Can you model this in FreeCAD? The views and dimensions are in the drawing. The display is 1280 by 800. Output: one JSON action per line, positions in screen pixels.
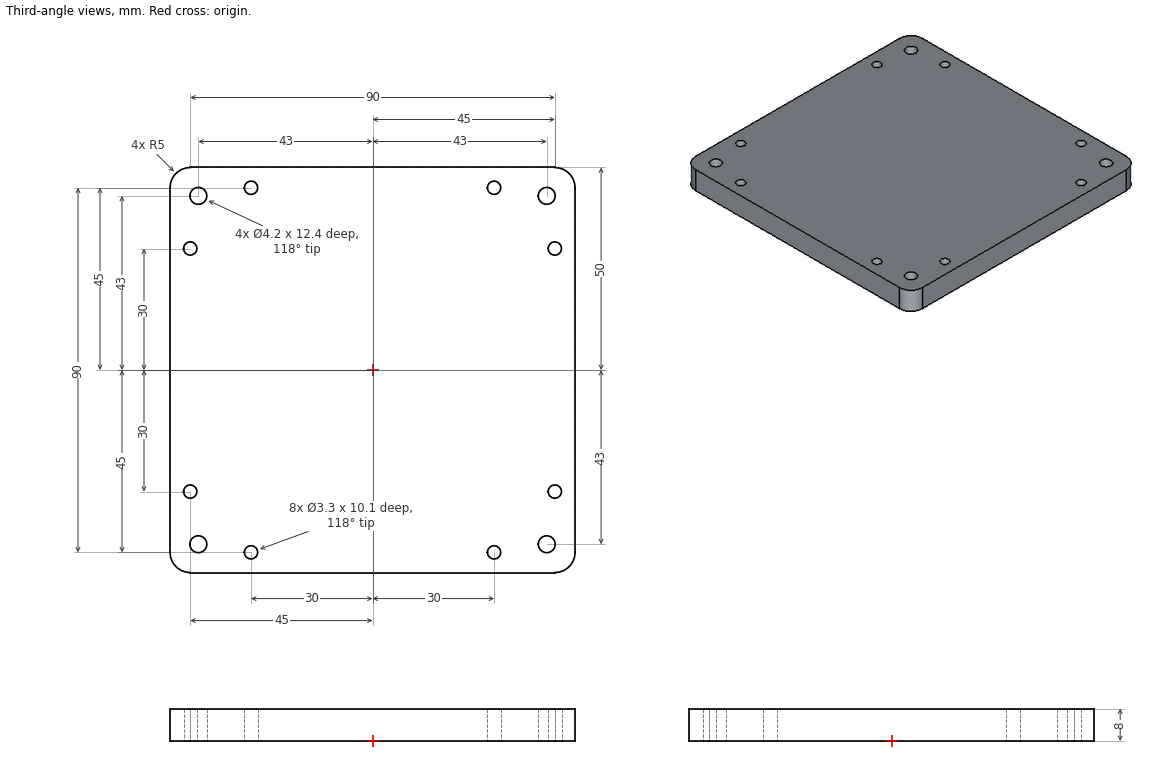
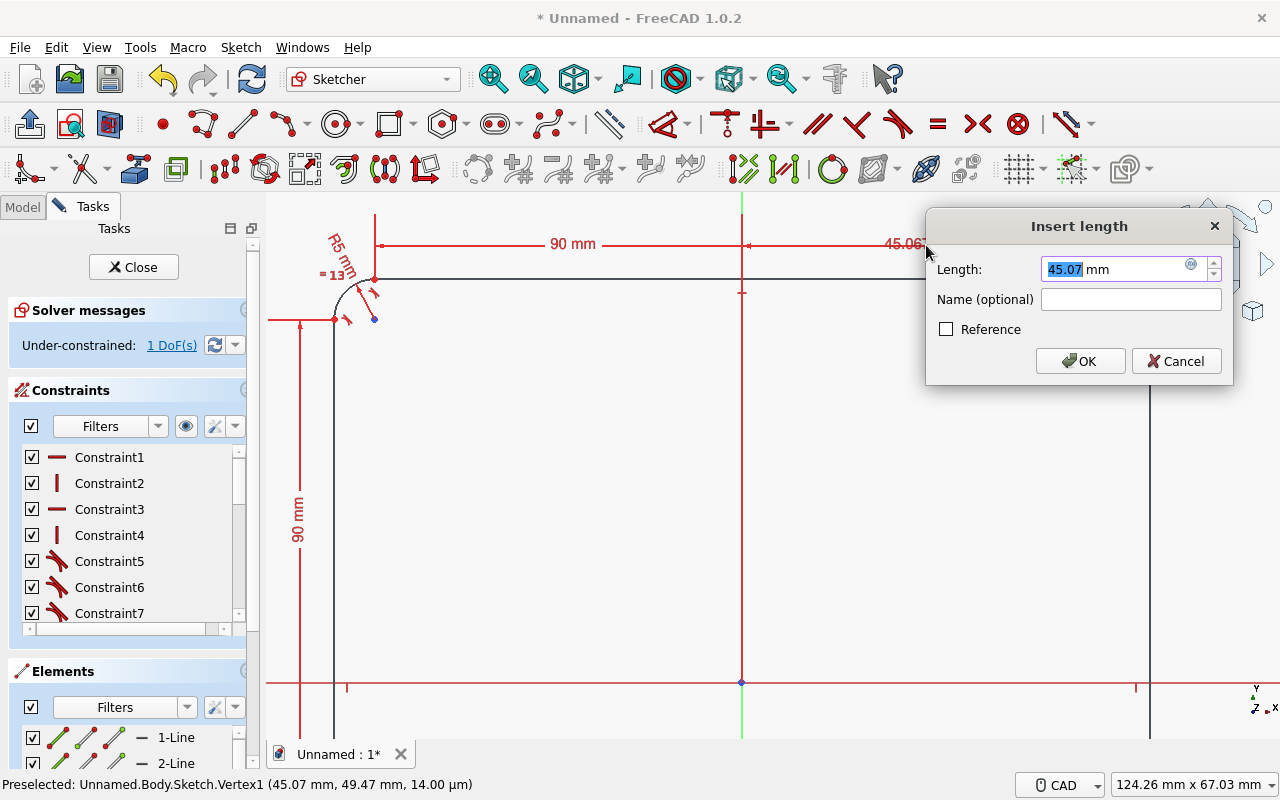
{"action": "type", "text": "45"}
{"action": "key", "text": "Return"}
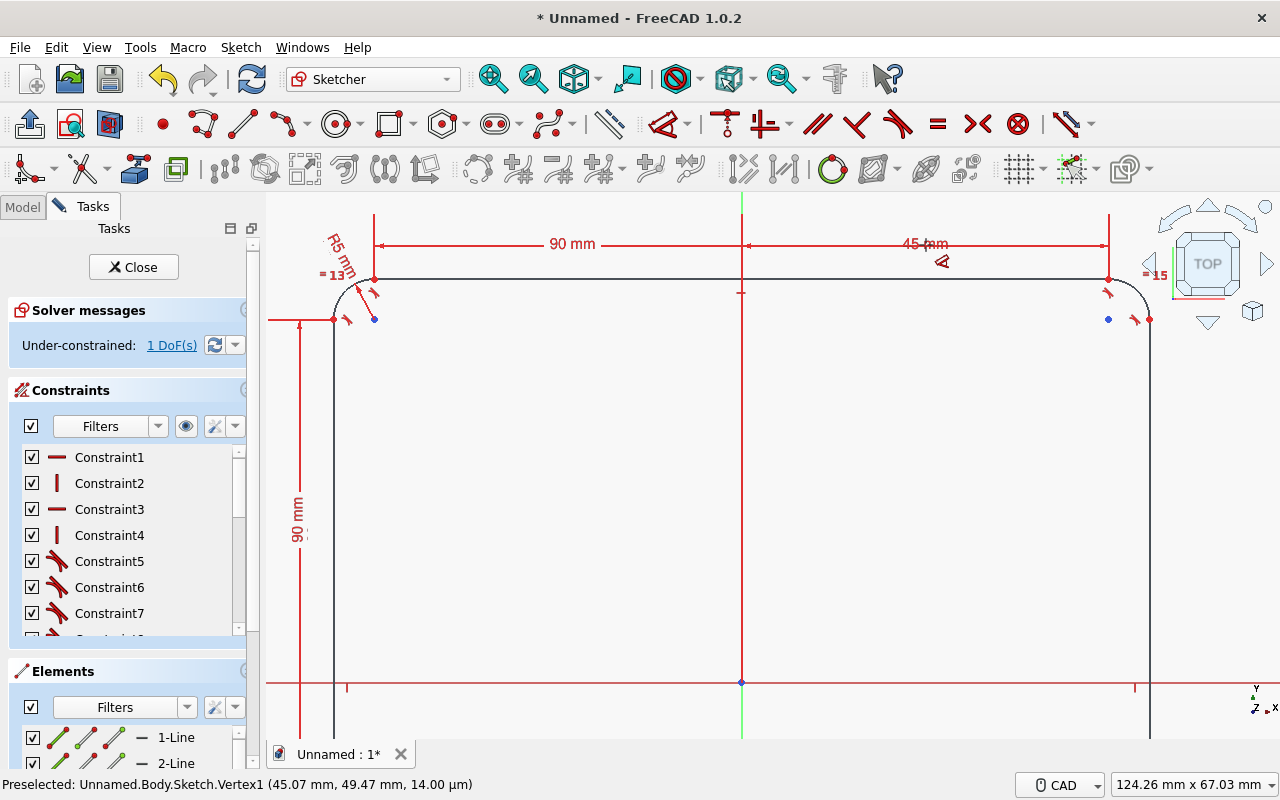
{"action": "left_click", "coordinate": [1109, 279]}
{"action": "left_click", "coordinate": [708, 481]}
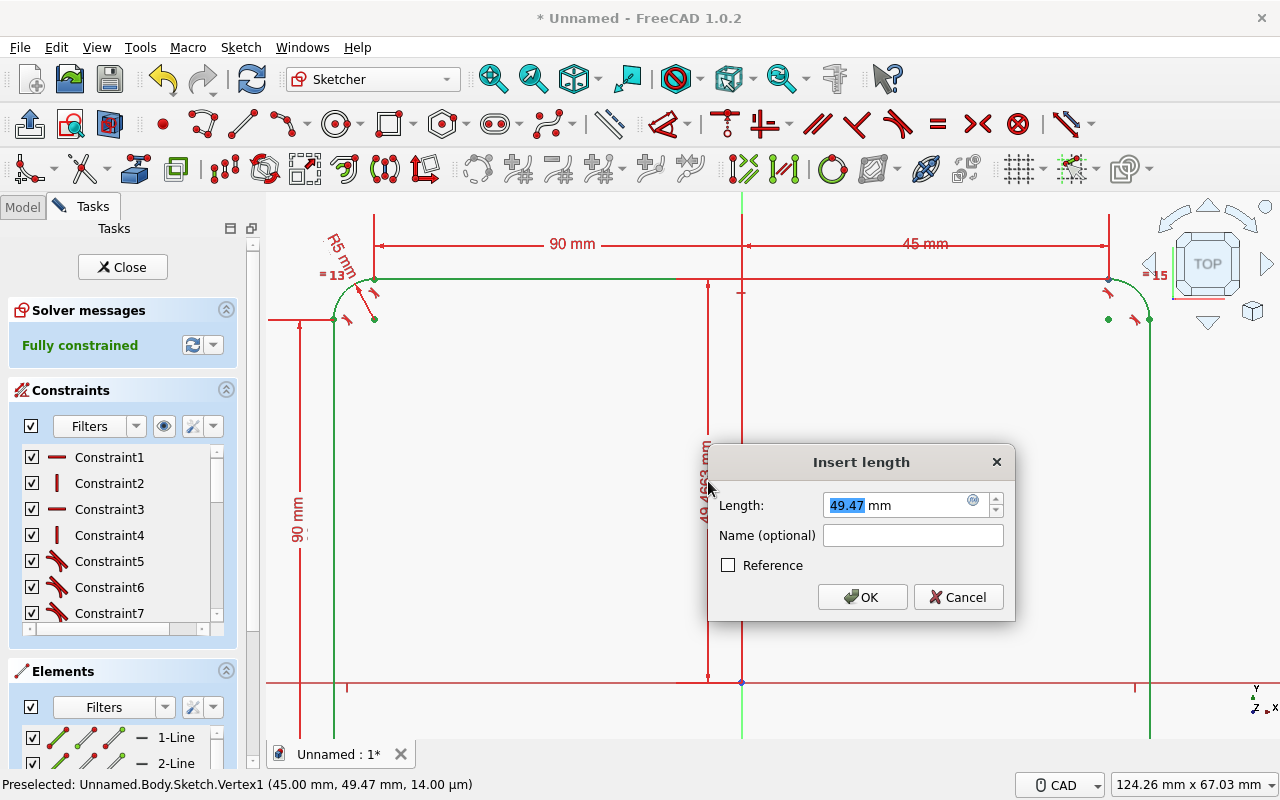
{"action": "type", "text": "50"}
{"action": "key", "text": "Return"}
{"action": "key", "text": "Escape"}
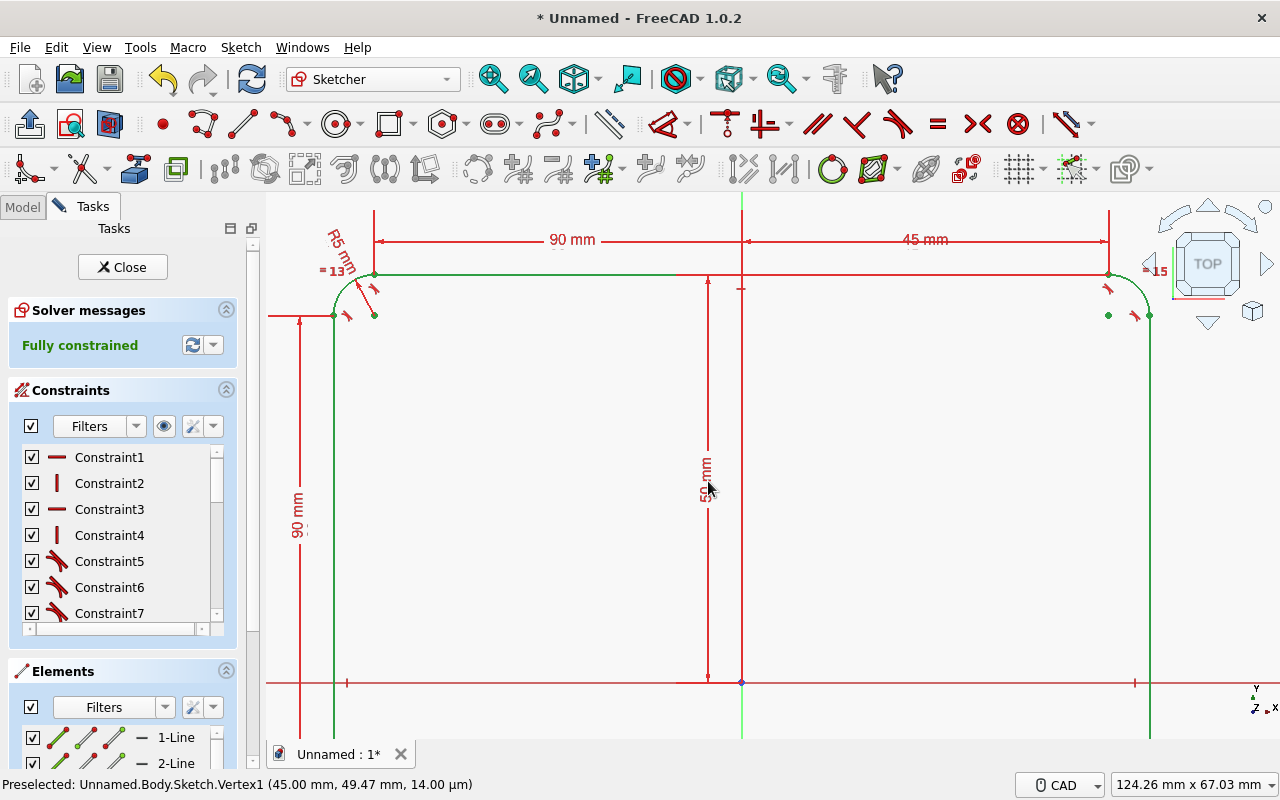
{"action": "left_click", "coordinate": [123, 267]}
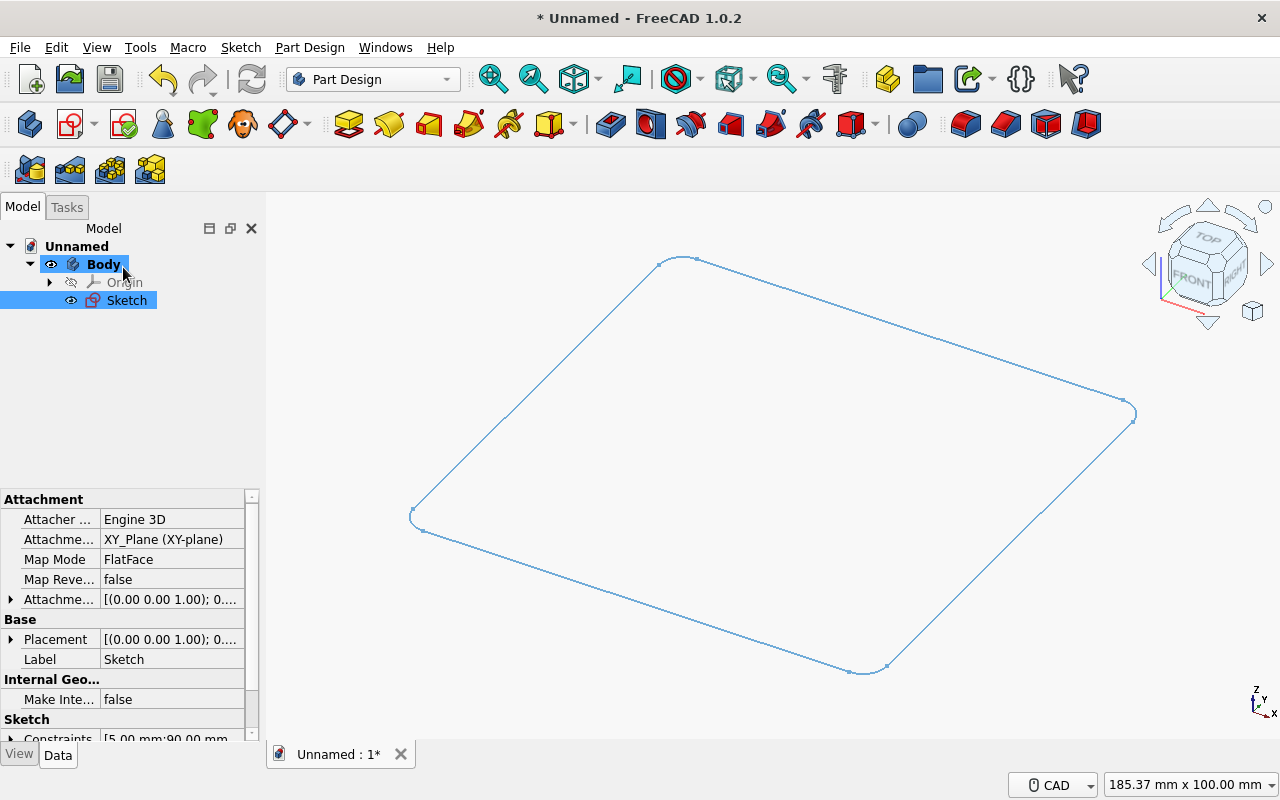
{"action": "left_click", "coordinate": [350, 124]}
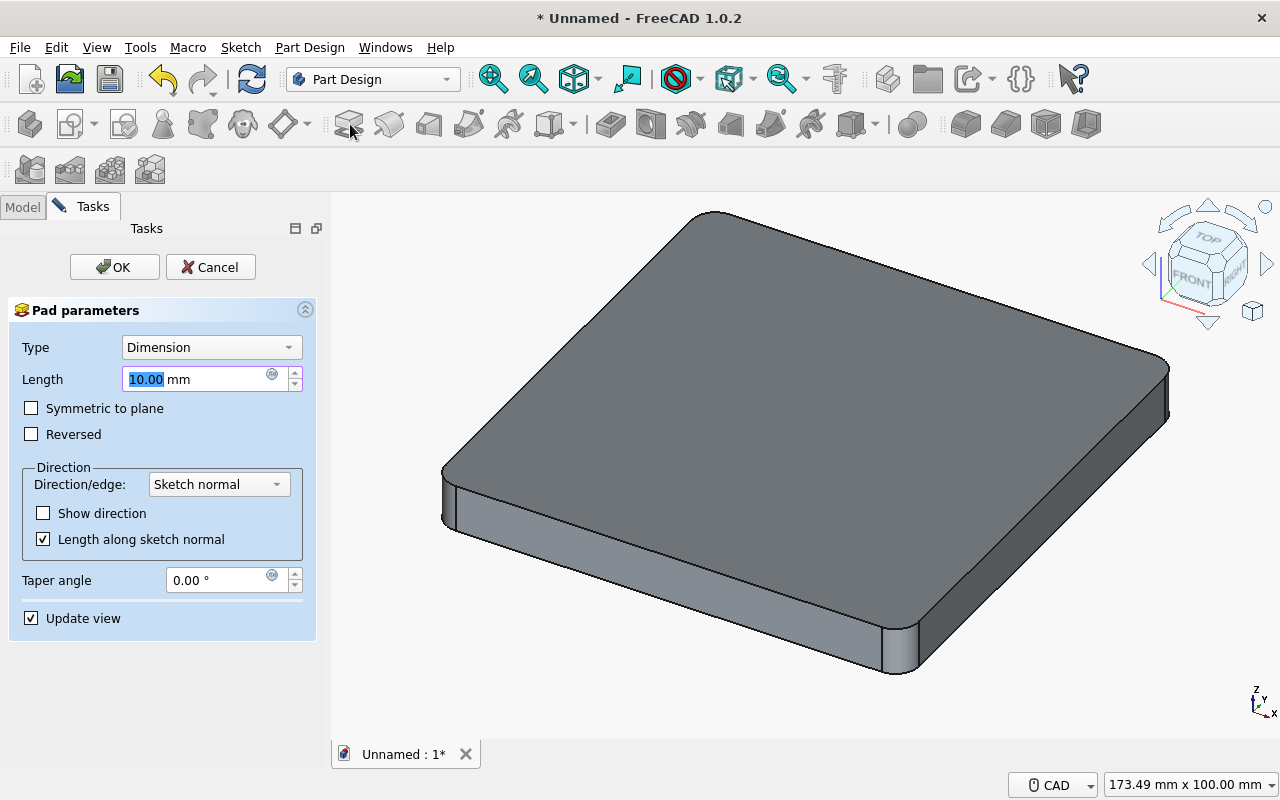
{"action": "type", "text": "8"}
{"action": "key", "text": "Tab"}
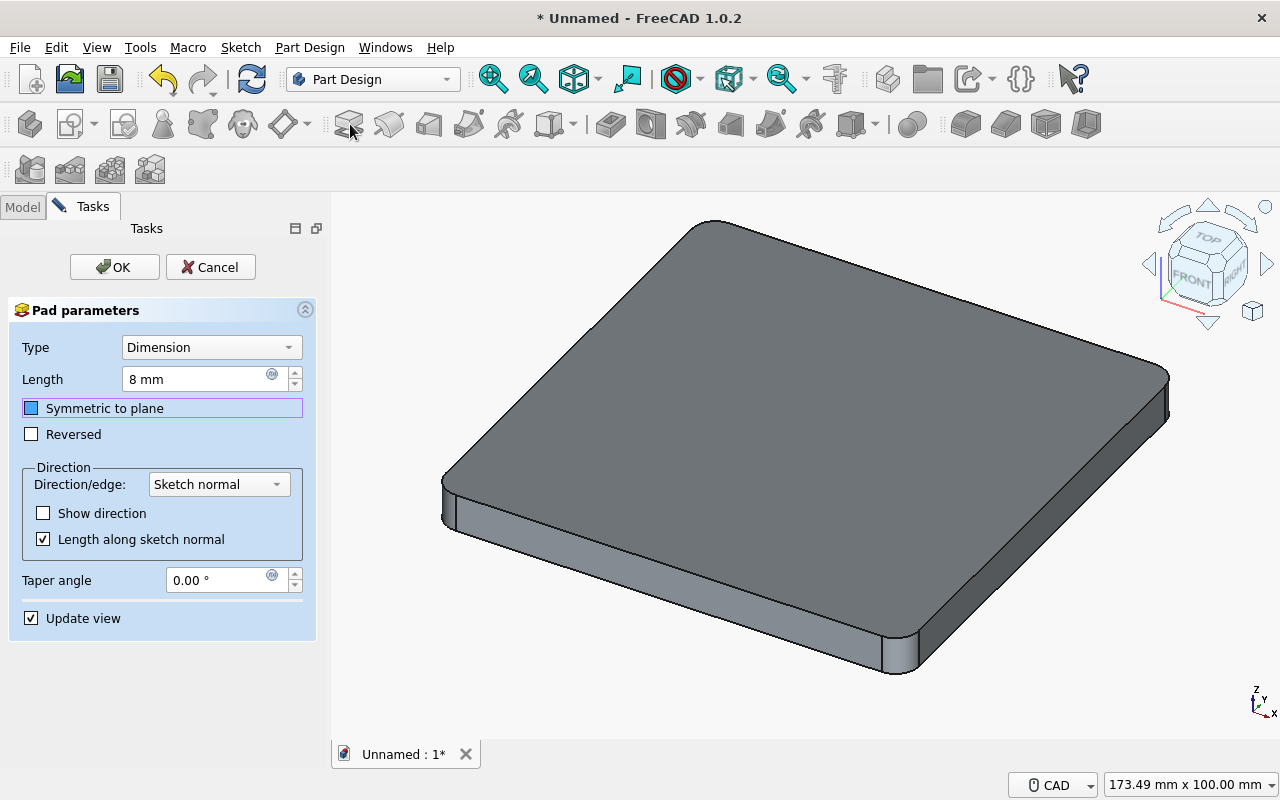
{"action": "left_click", "coordinate": [115, 267]}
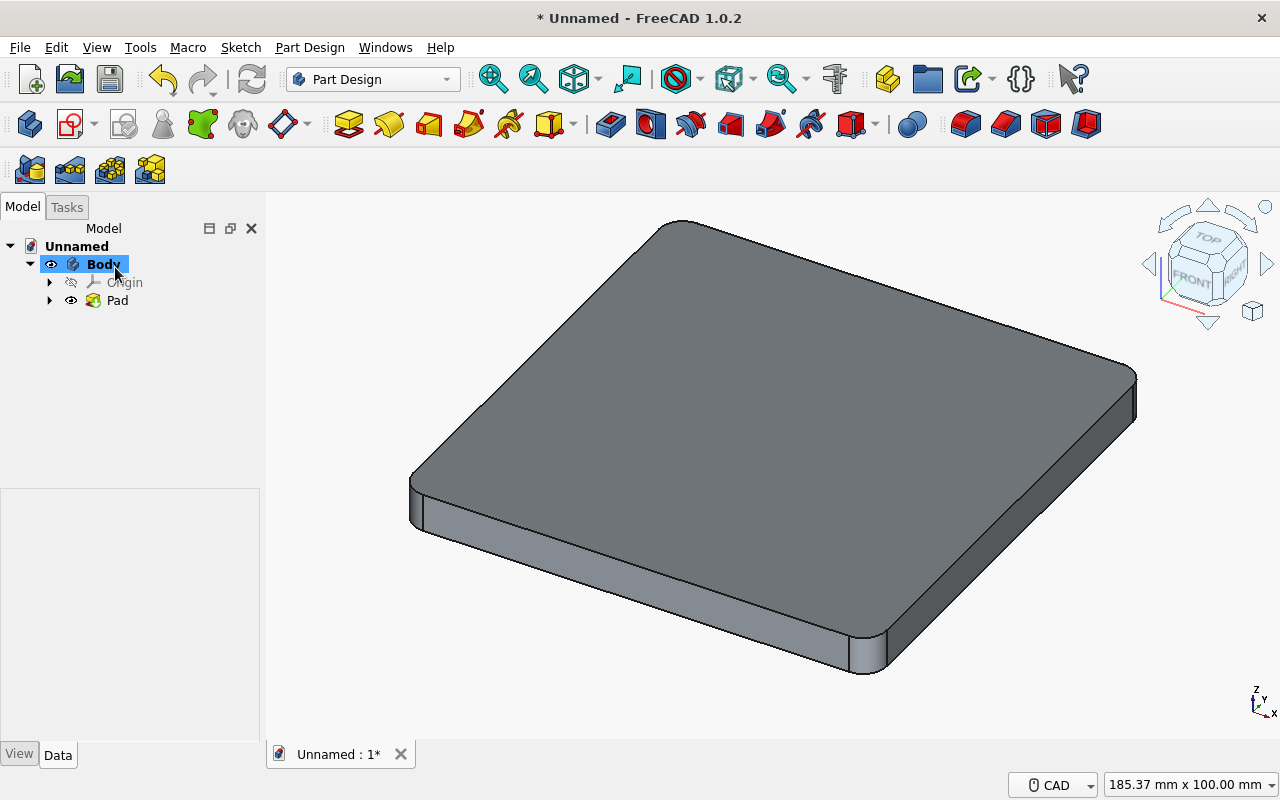
{"action": "left_click", "coordinate": [773, 429]}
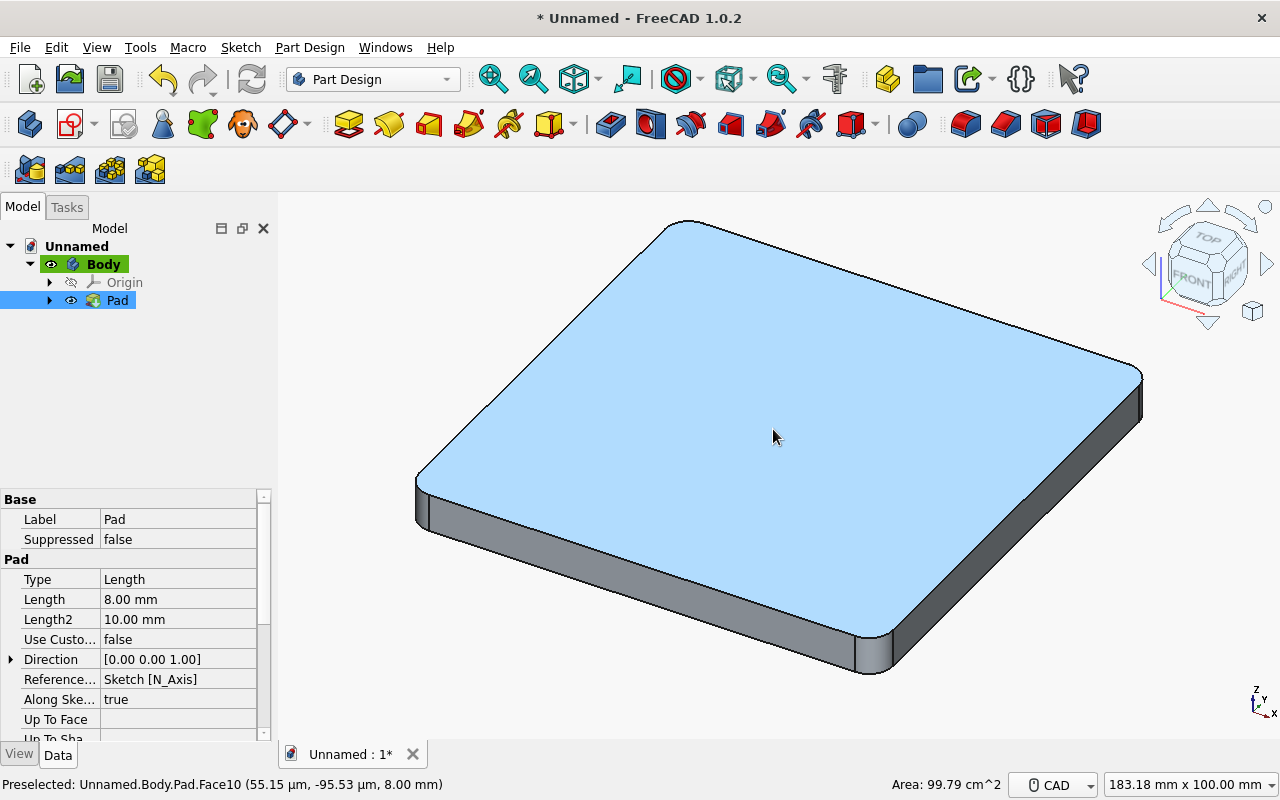
{"action": "left_click", "coordinate": [70, 124]}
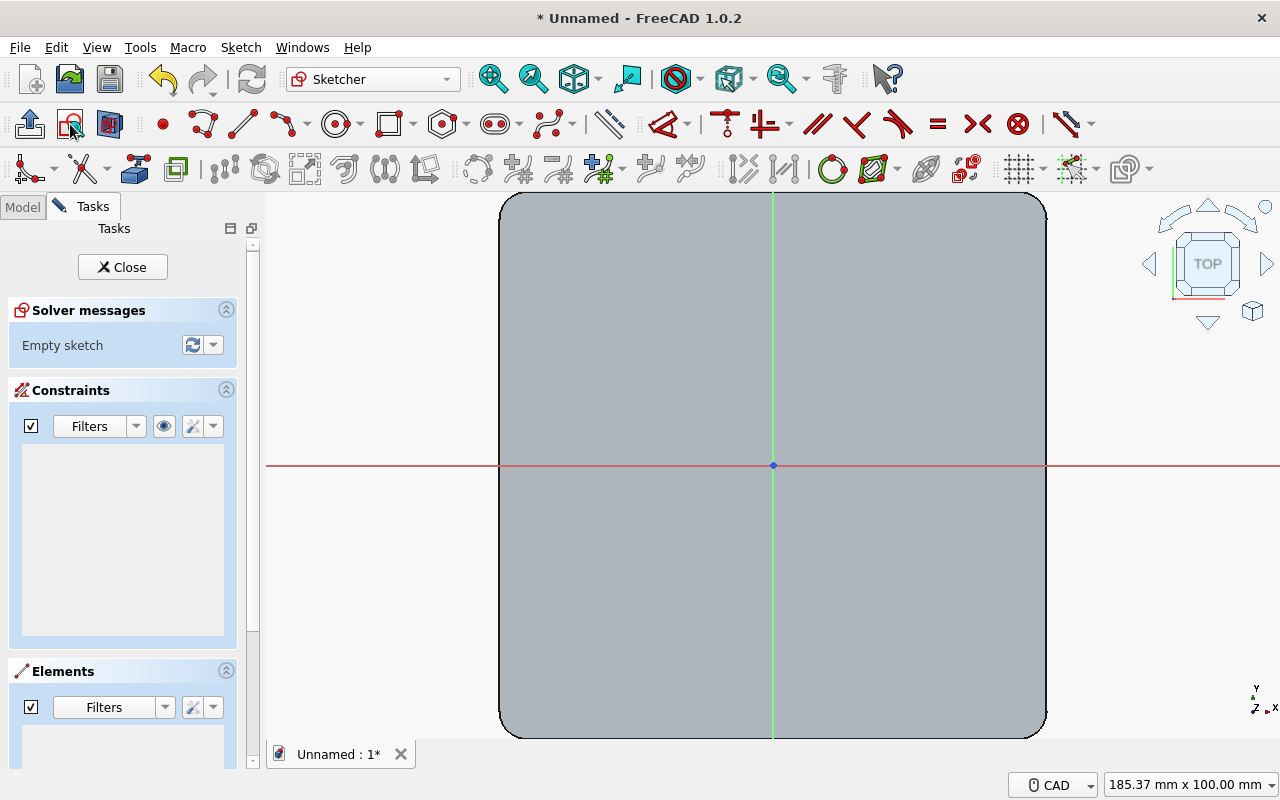
{"action": "scroll", "coordinate": [565, 466], "scroll_direction": "down", "scroll_amount": 2}